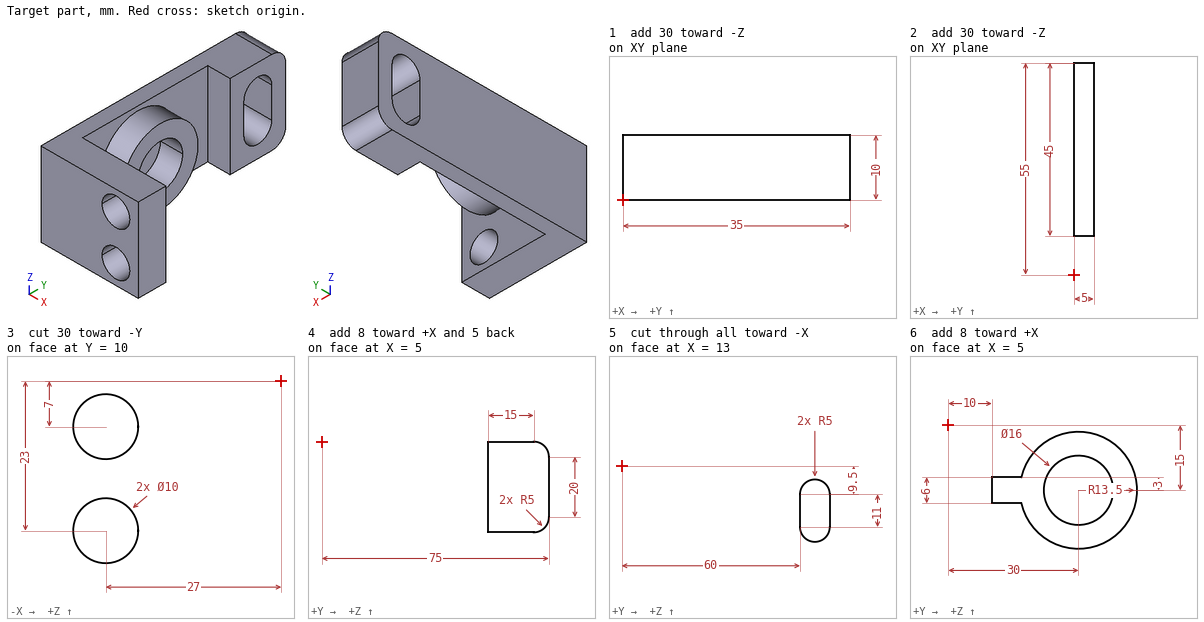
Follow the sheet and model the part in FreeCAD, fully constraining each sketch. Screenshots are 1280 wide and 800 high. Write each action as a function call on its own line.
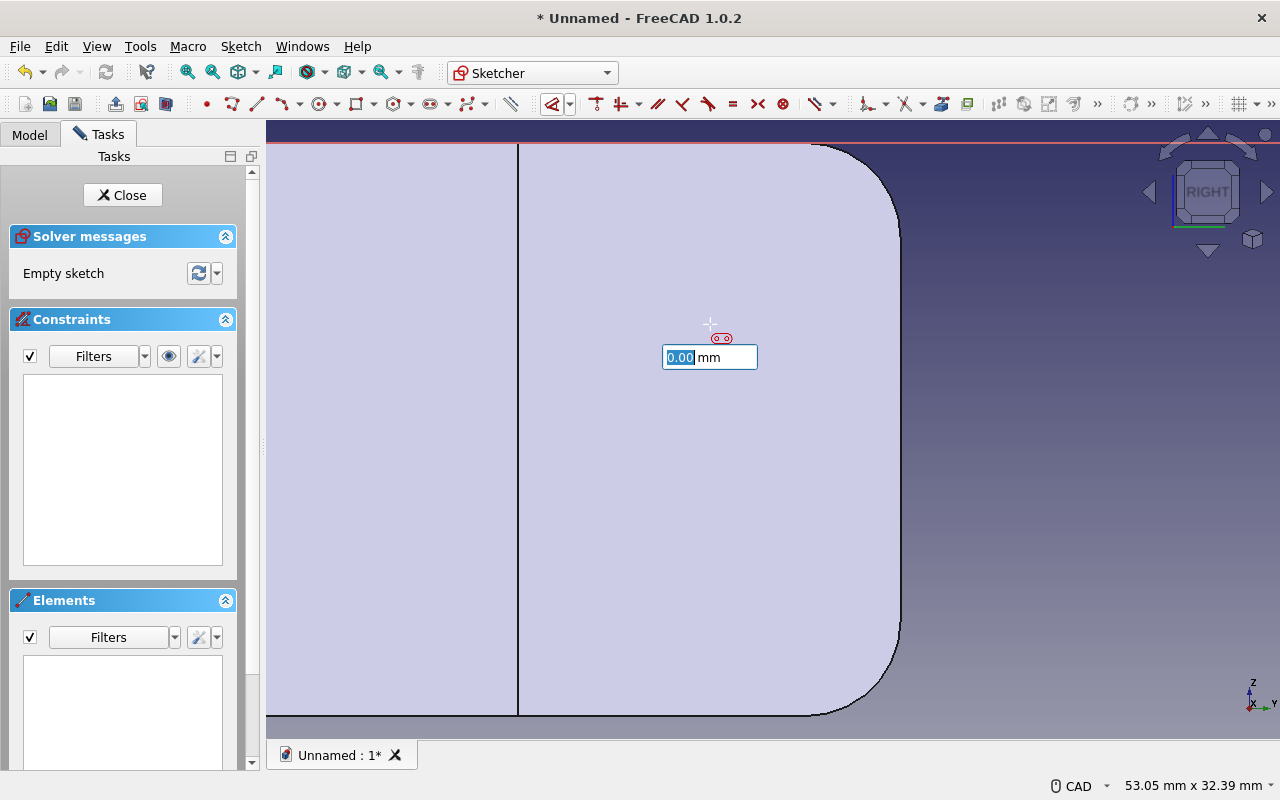
click(805, 430)
key(Escape)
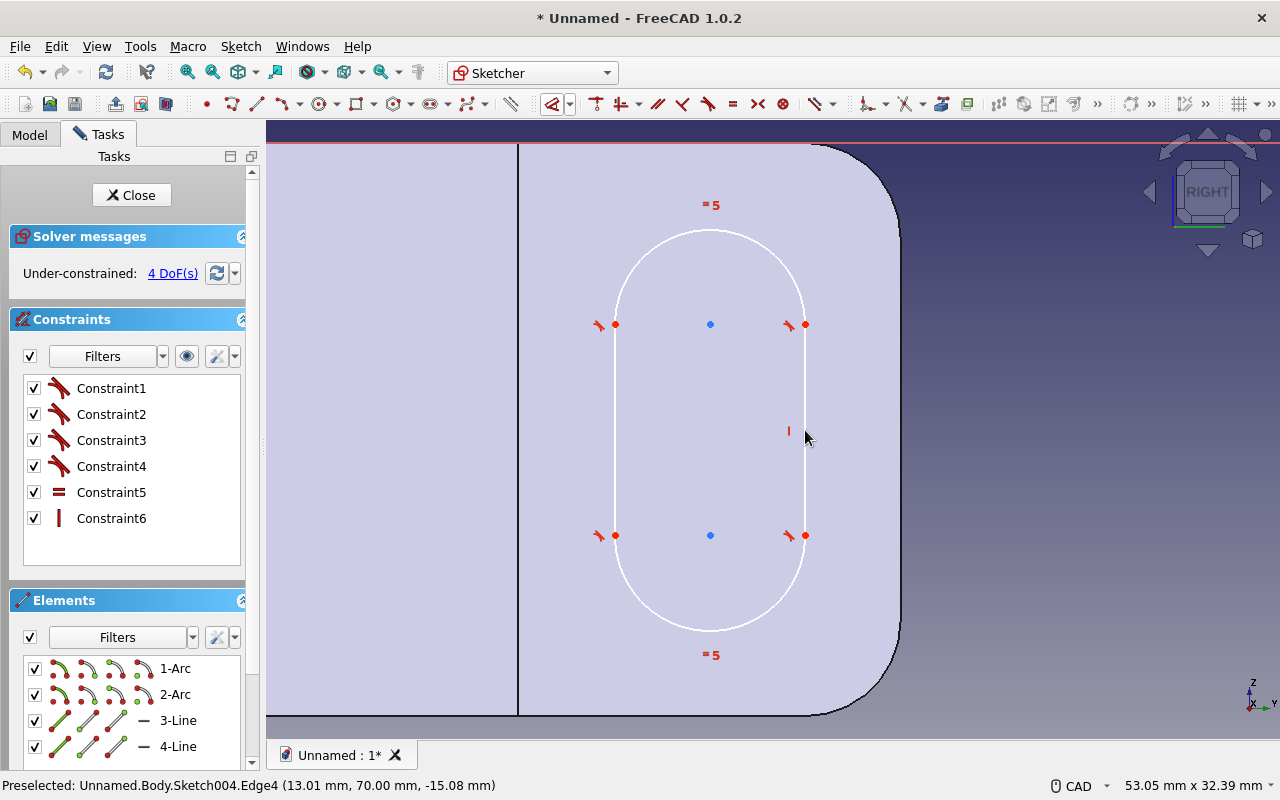
key(d)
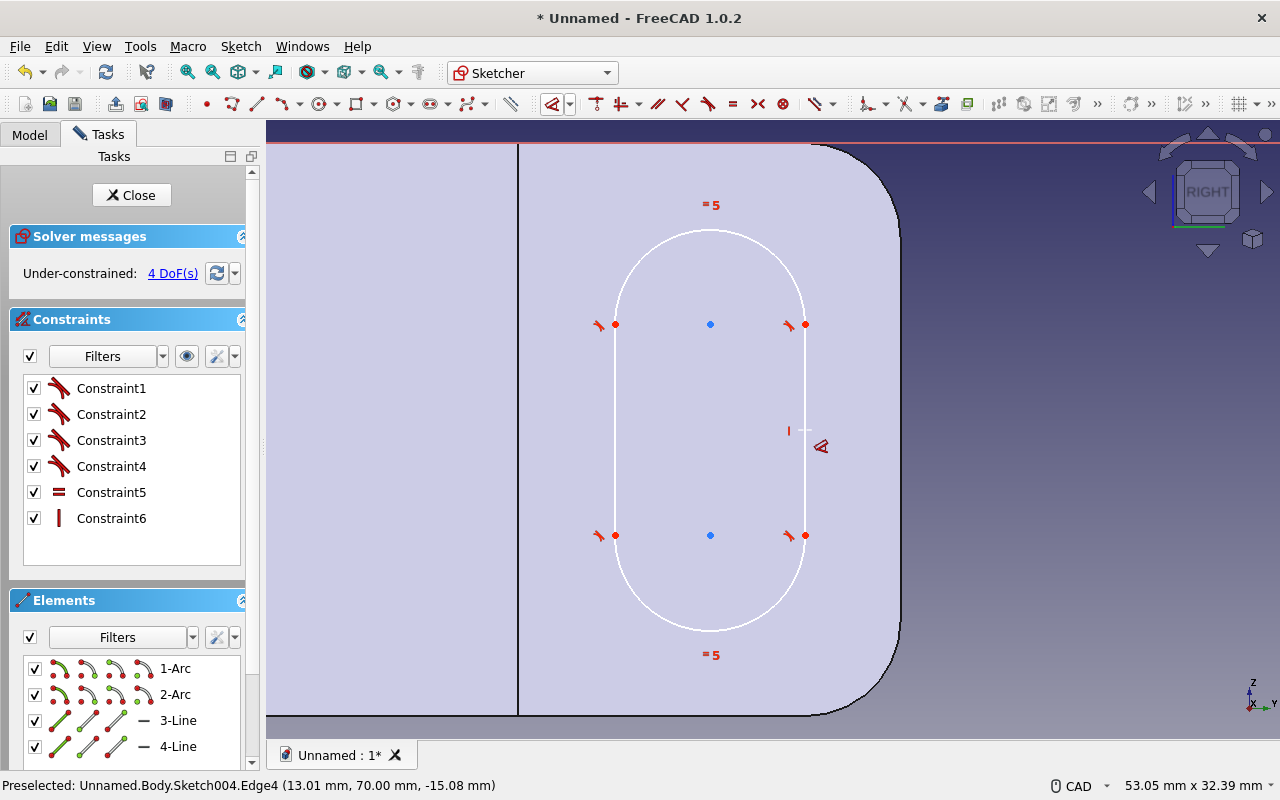
click(654, 613)
click(635, 639)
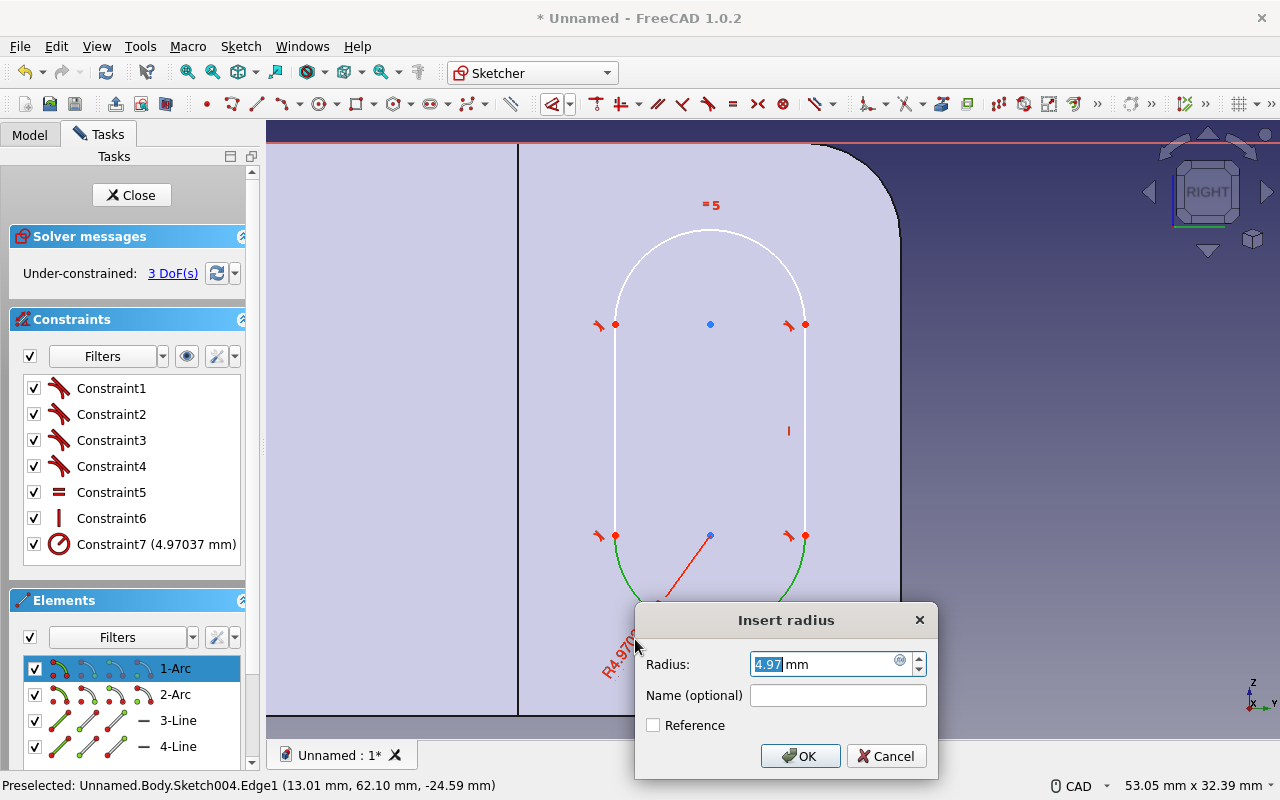
text(5)
key(Return)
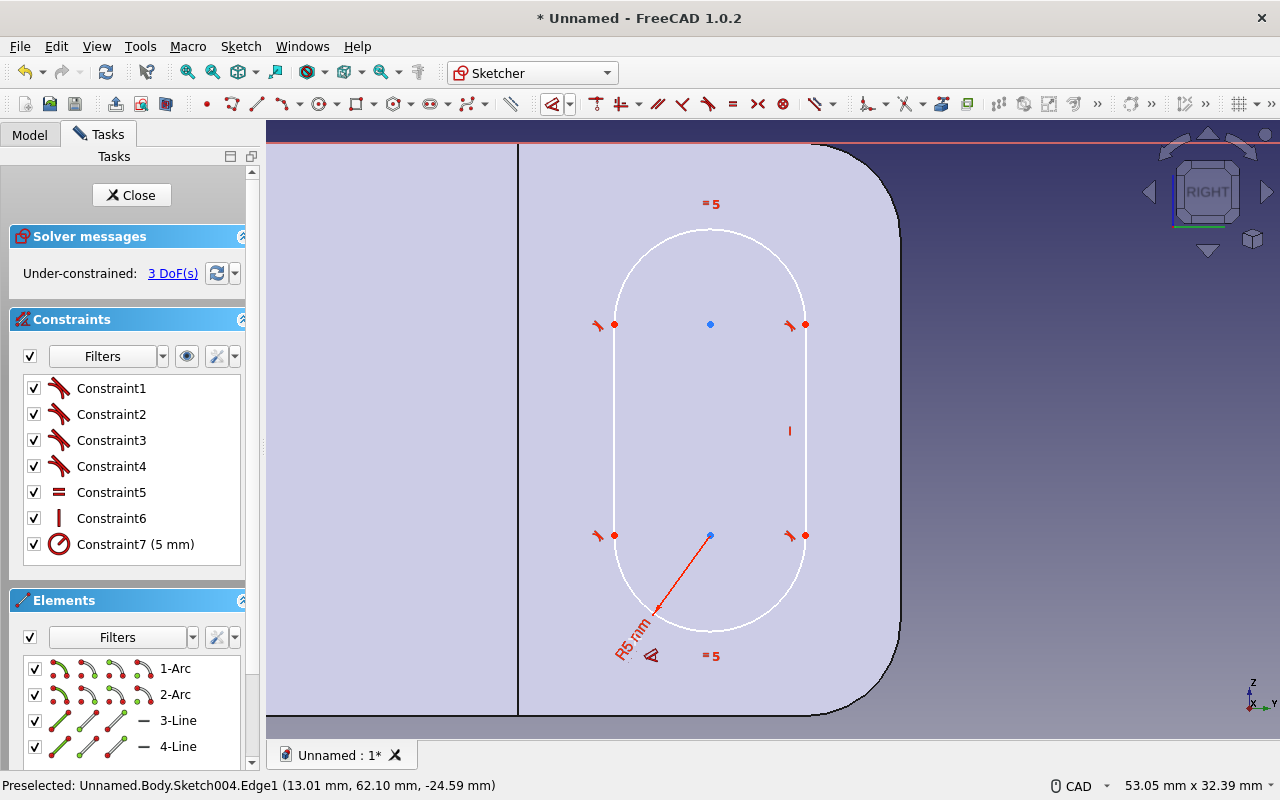
click(614, 473)
click(580, 431)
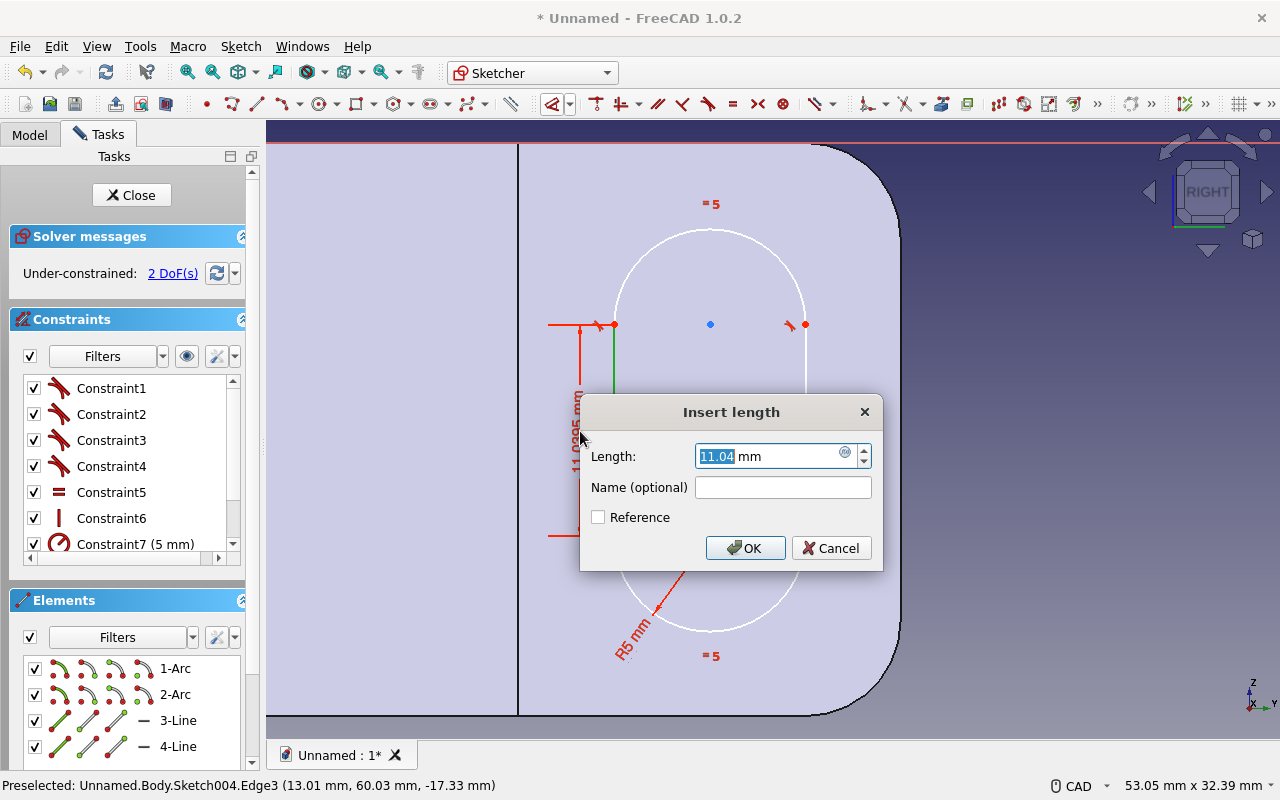
text(11)
key(Return)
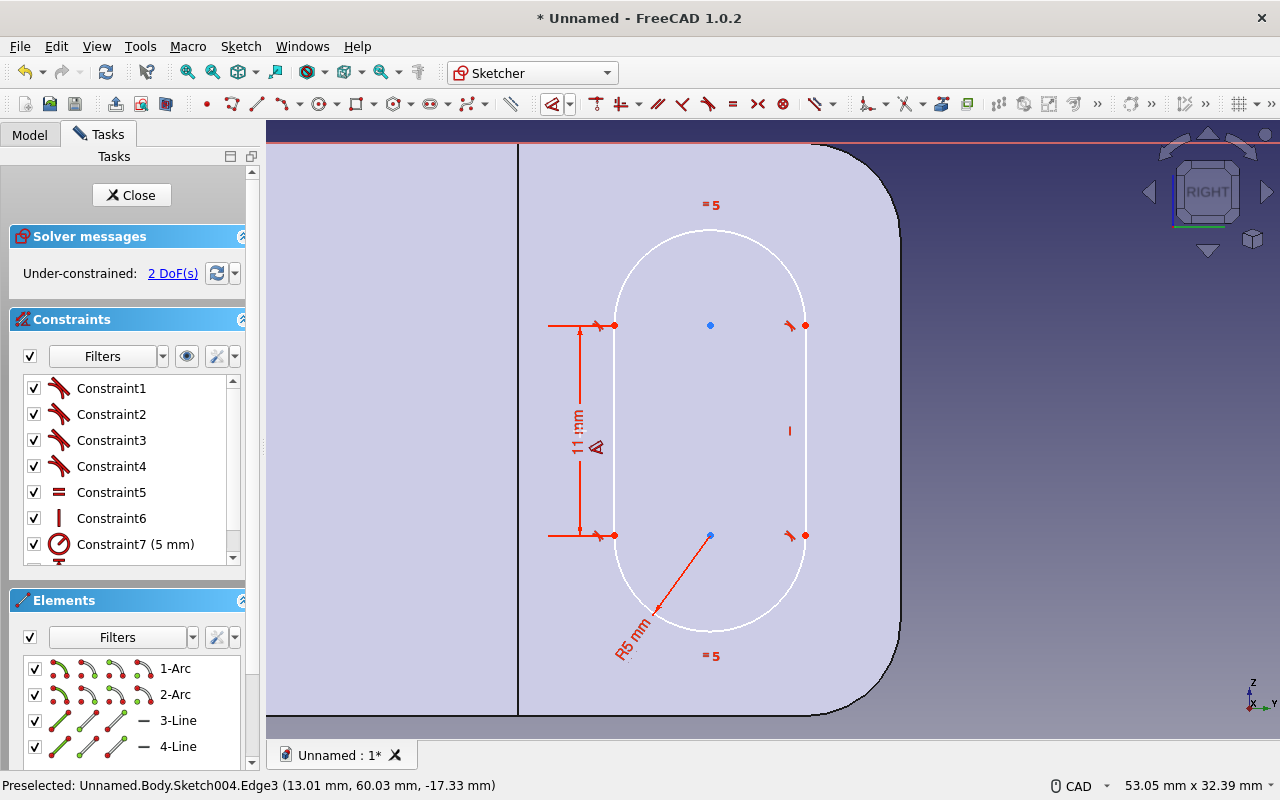
click(614, 536)
click(454, 570)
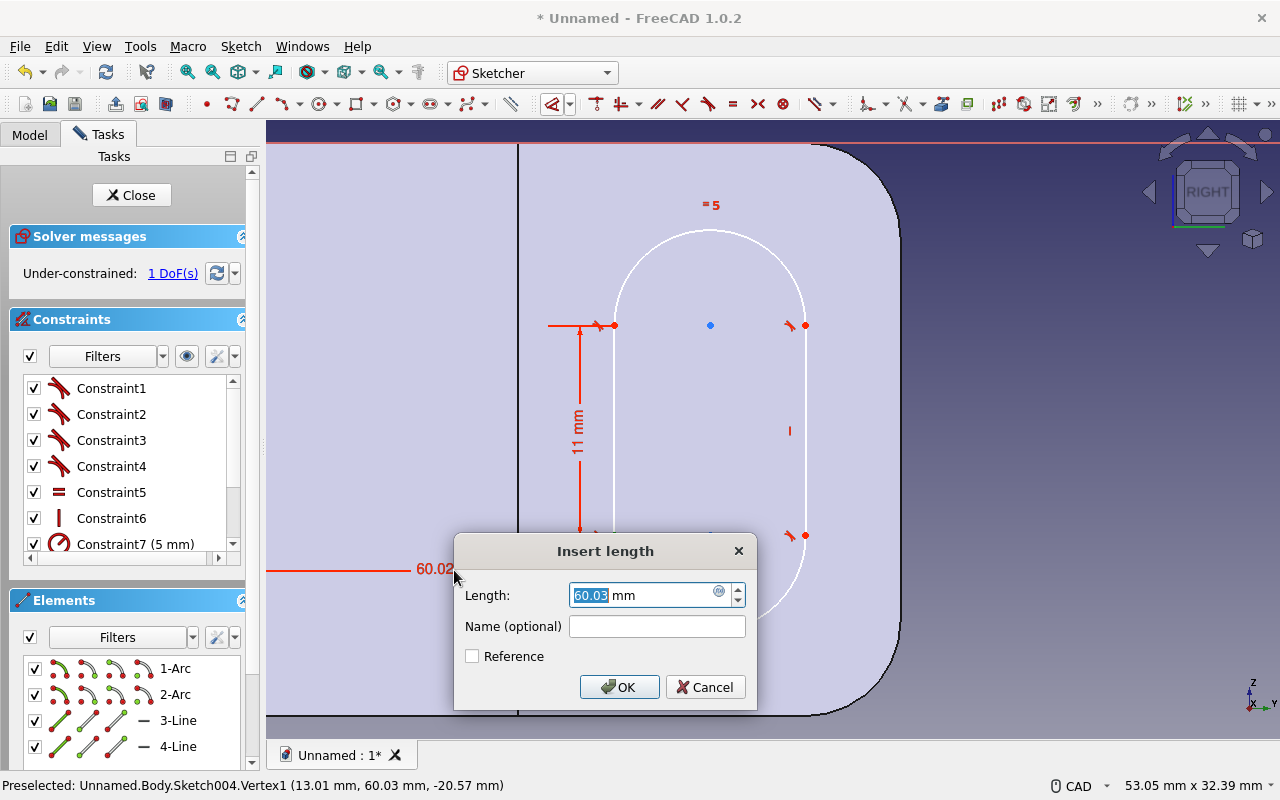
text(60)
key(Return)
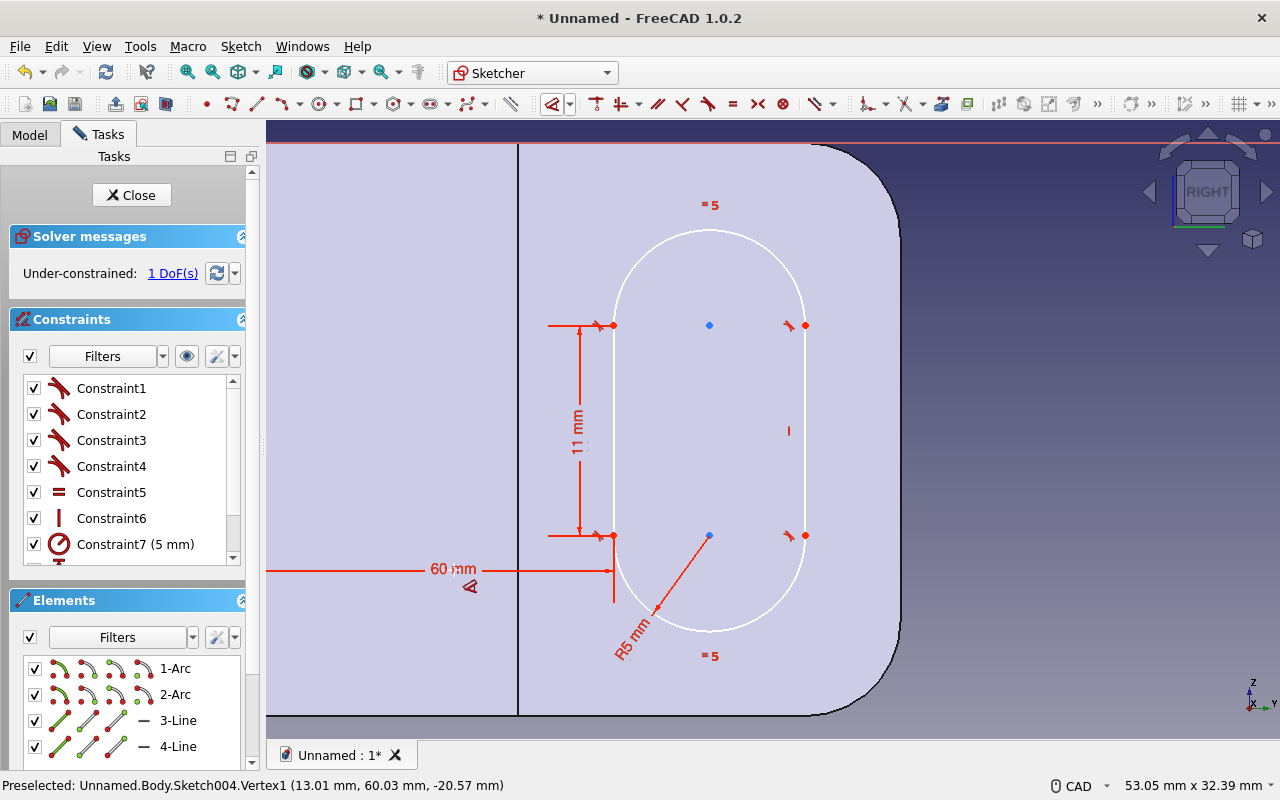
click(805, 326)
click(839, 237)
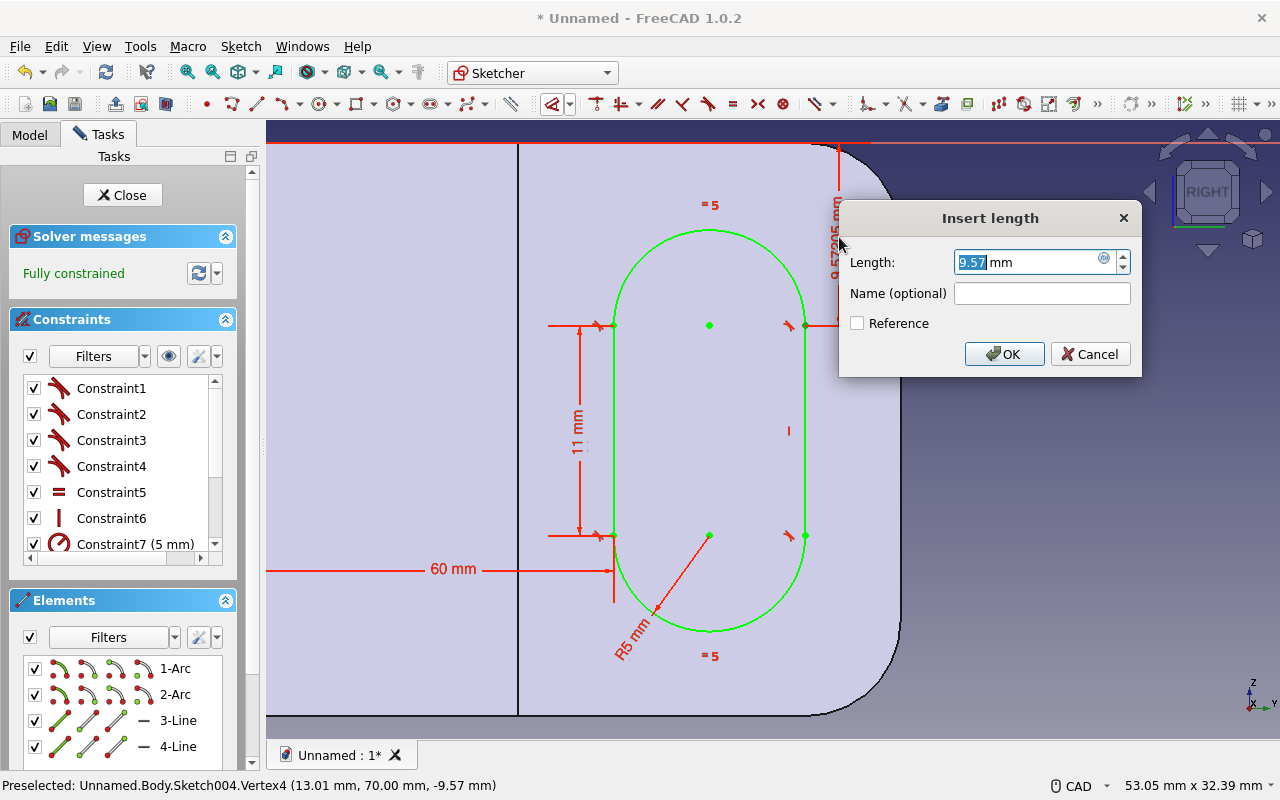
text(9.5)
key(Return)
key(Escape)